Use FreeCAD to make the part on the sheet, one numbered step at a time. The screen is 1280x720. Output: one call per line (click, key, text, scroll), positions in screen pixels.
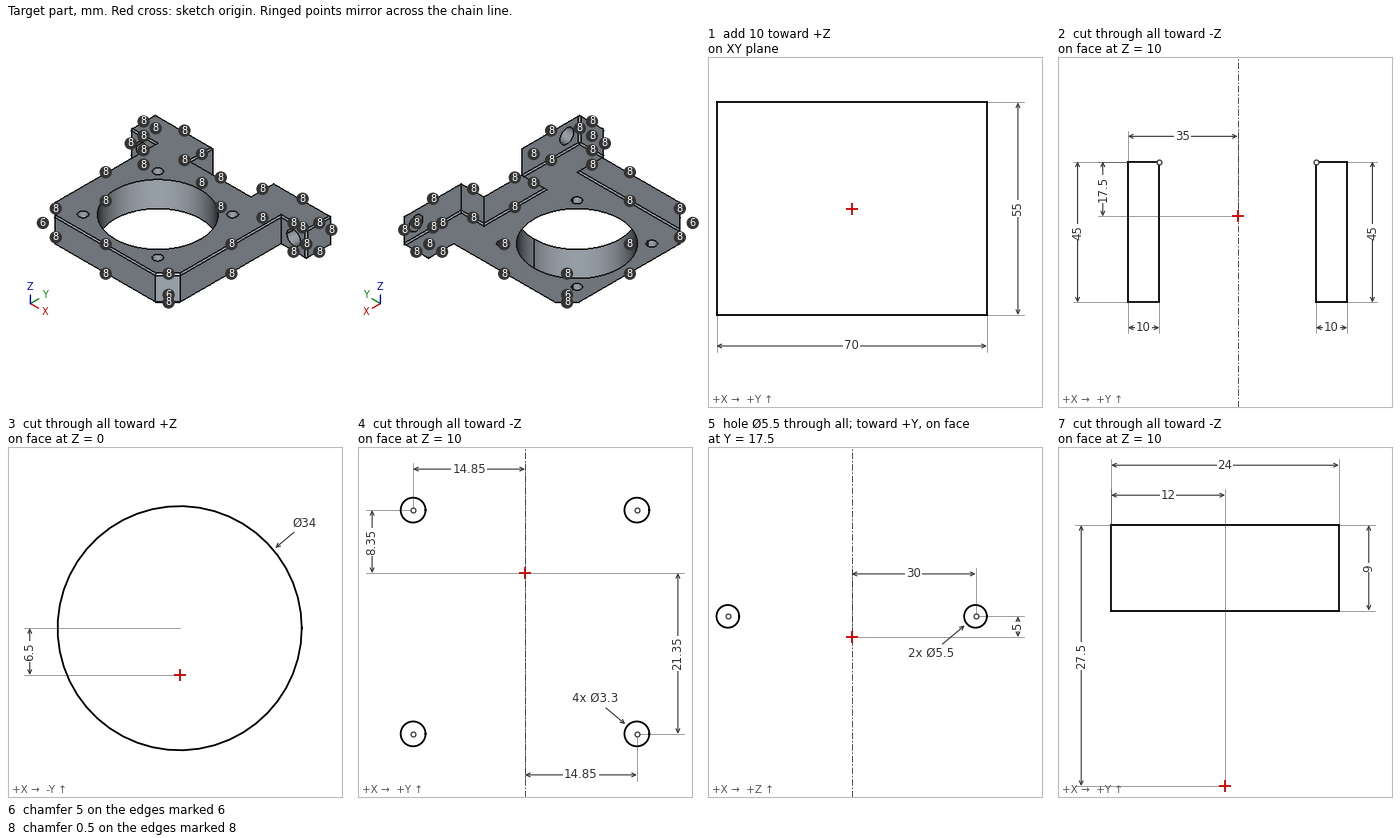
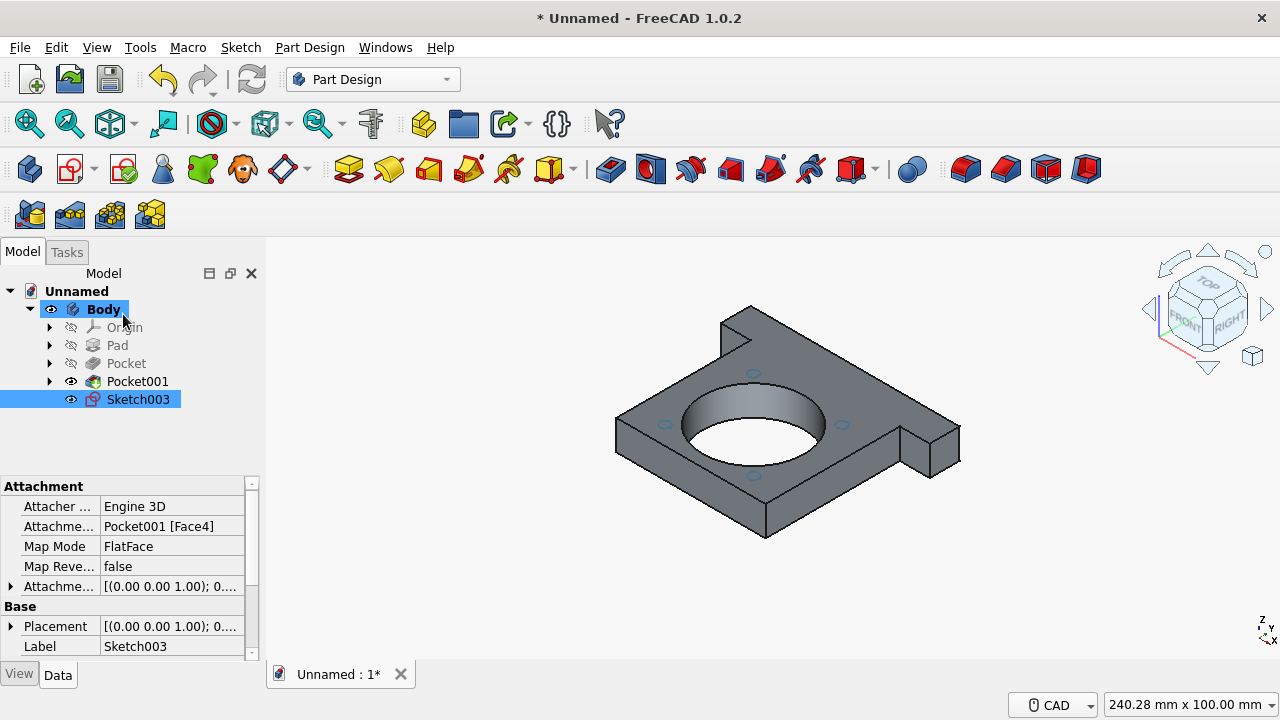
click(612, 170)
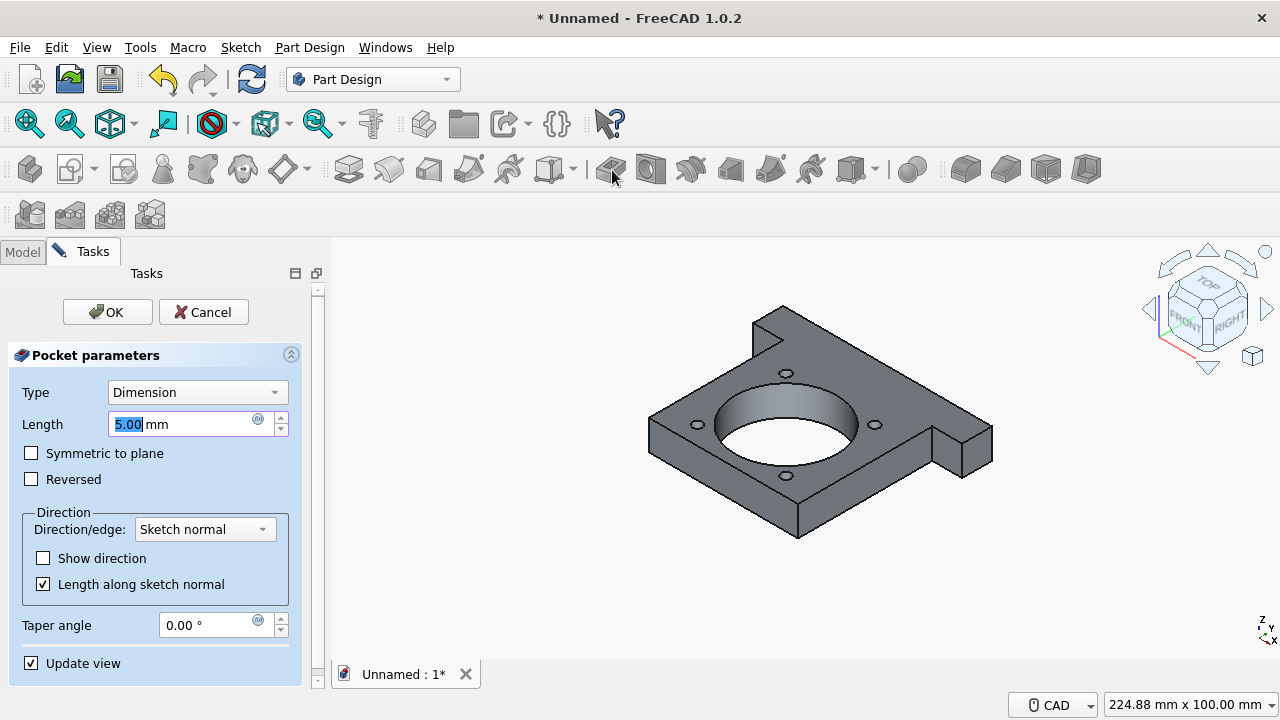
click(198, 392)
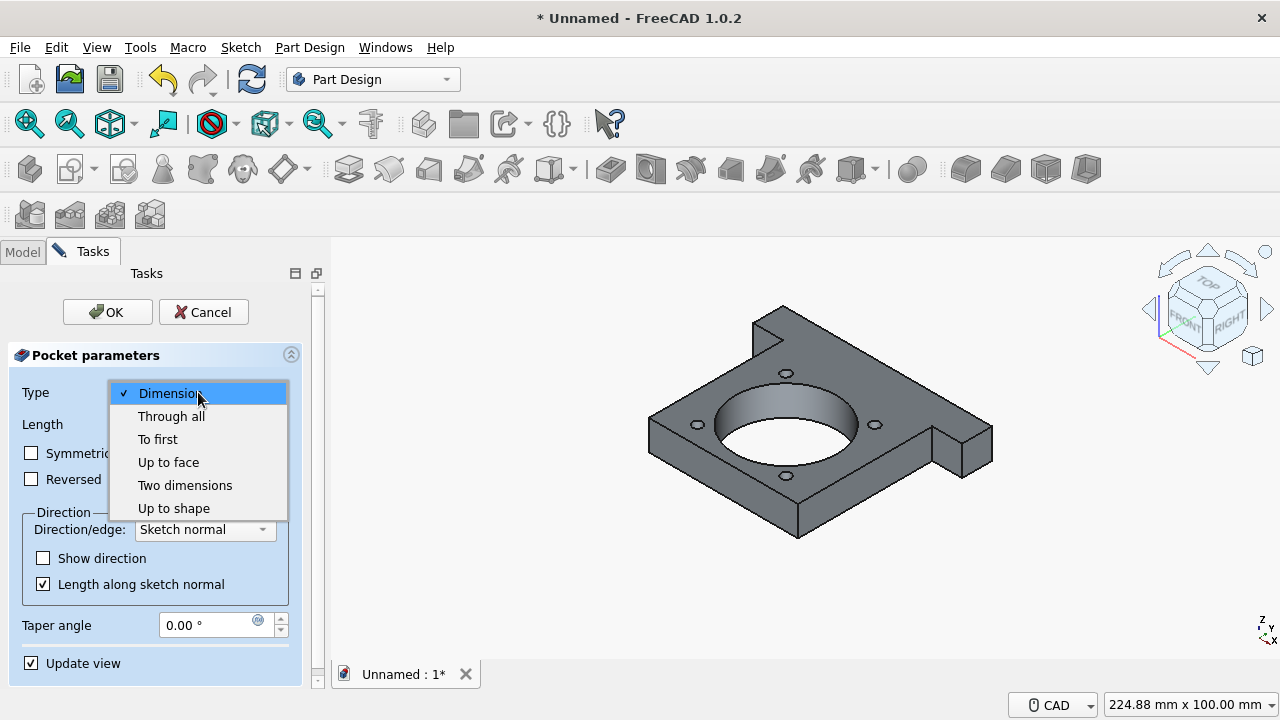
click(198, 416)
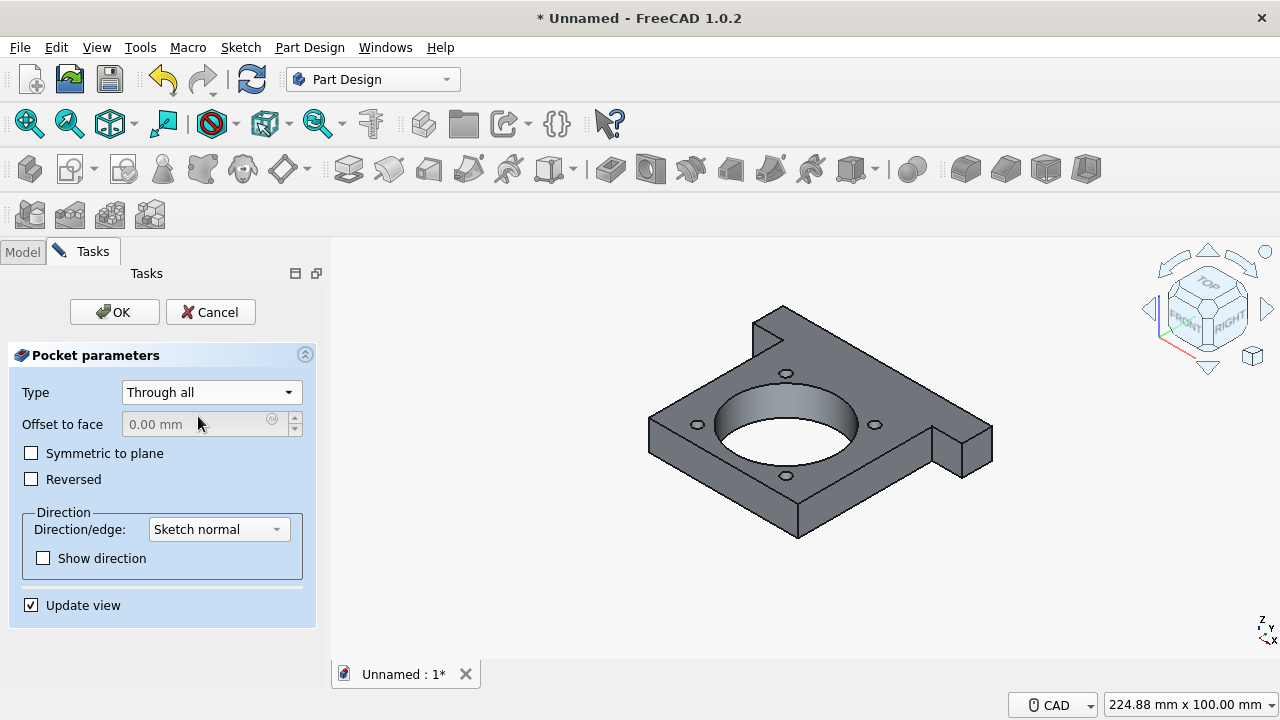
click(115, 312)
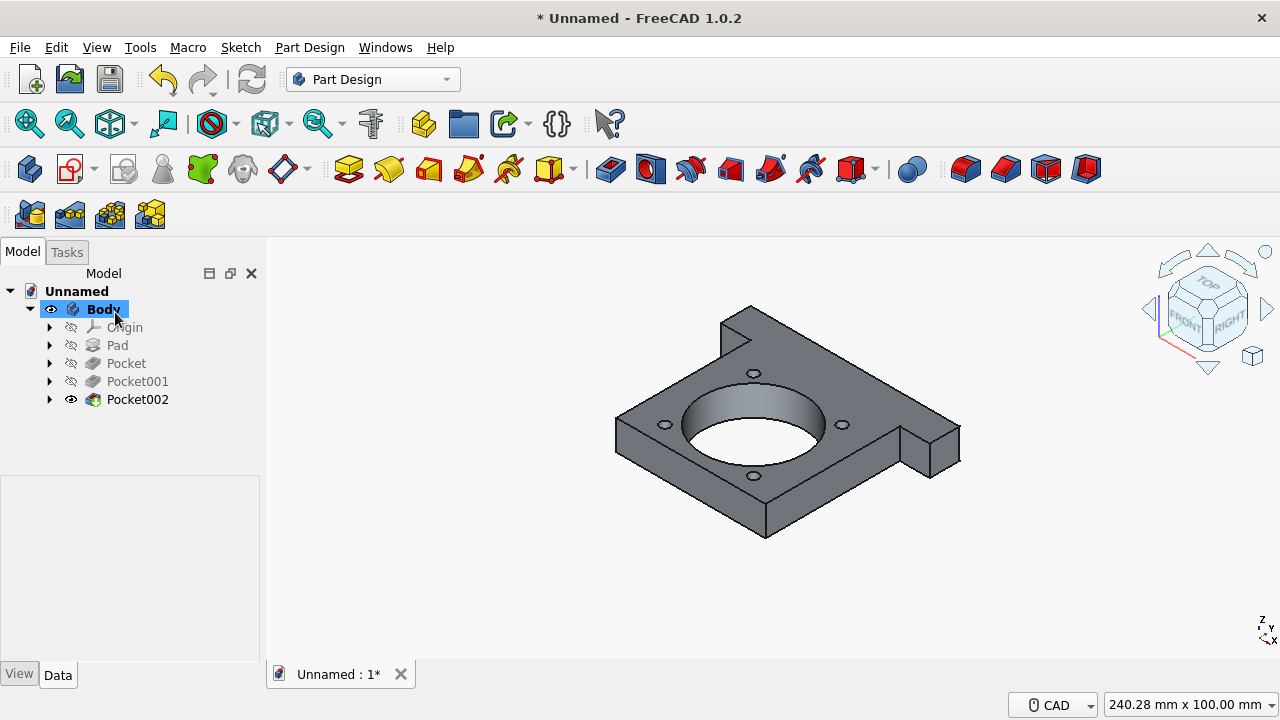
click(915, 451)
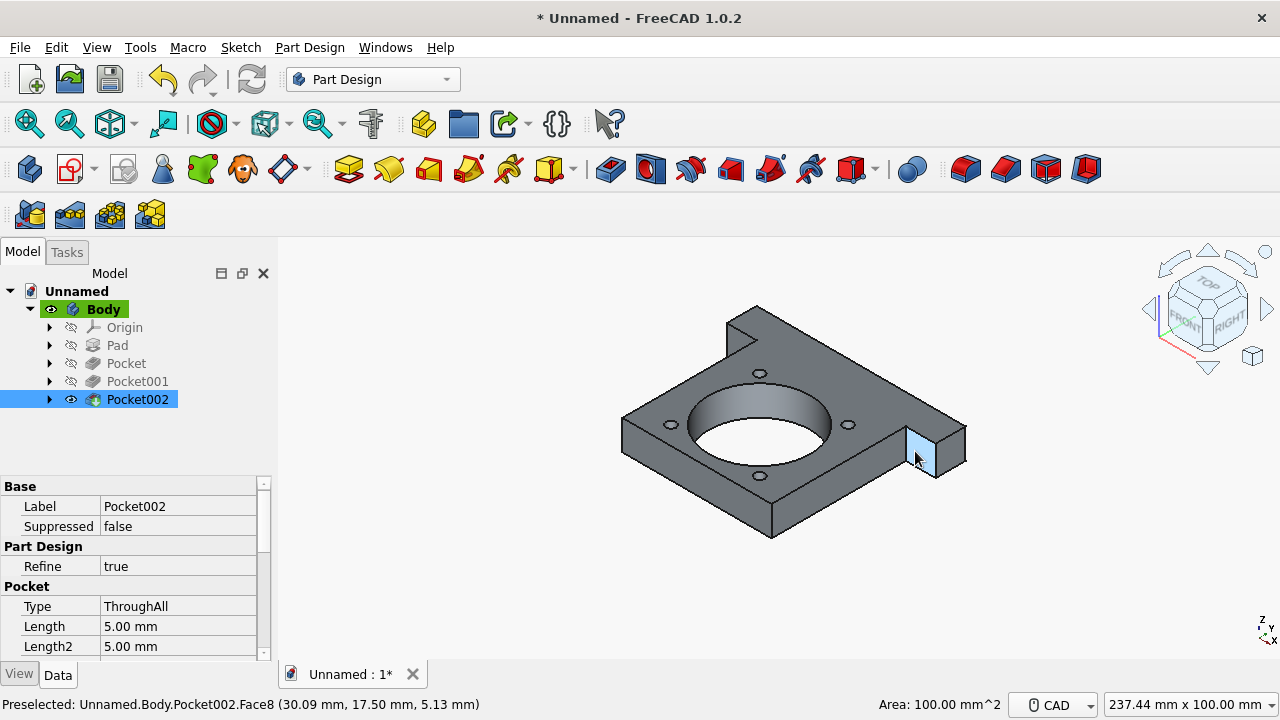
click(70, 170)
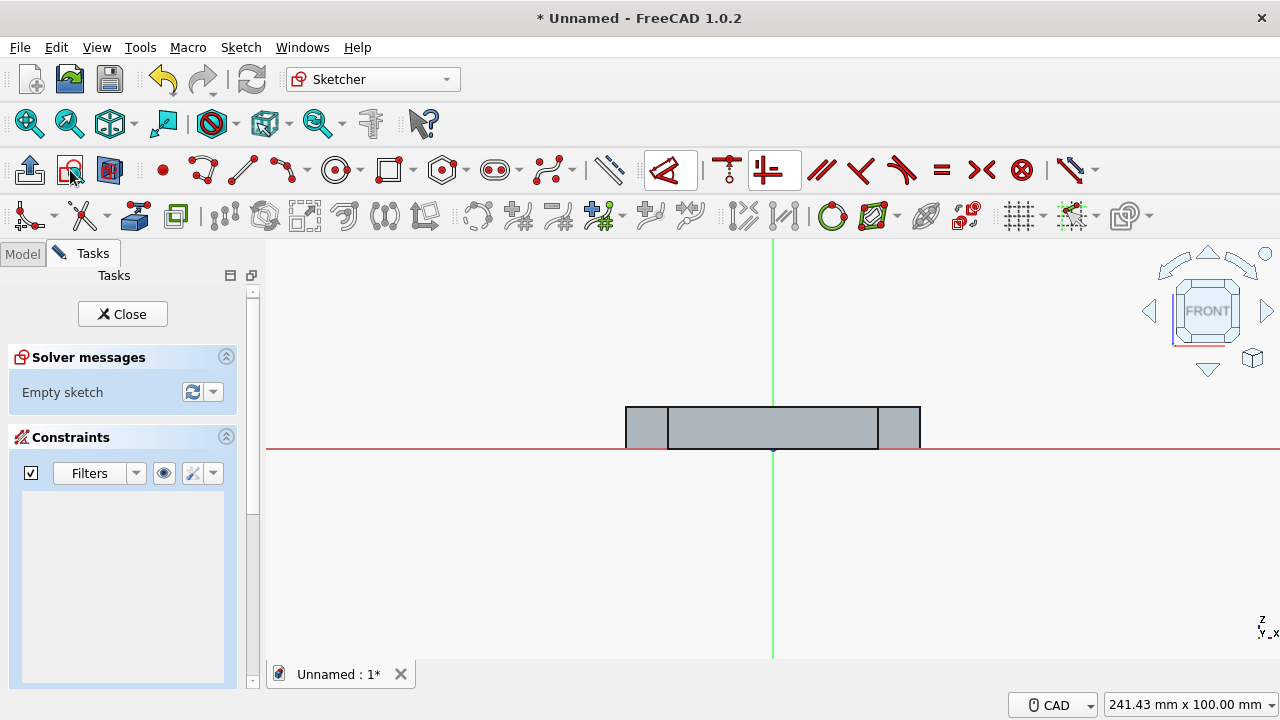
scroll(829, 419, up, 4)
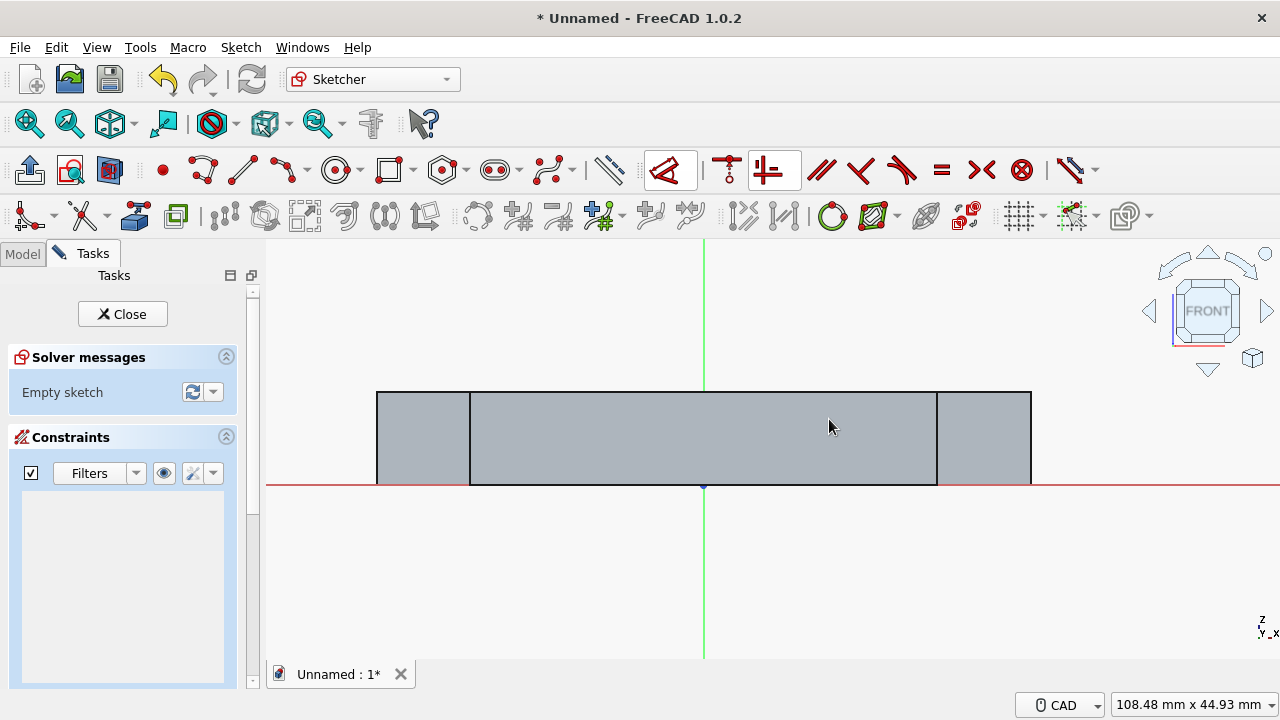
key(g)
key(c)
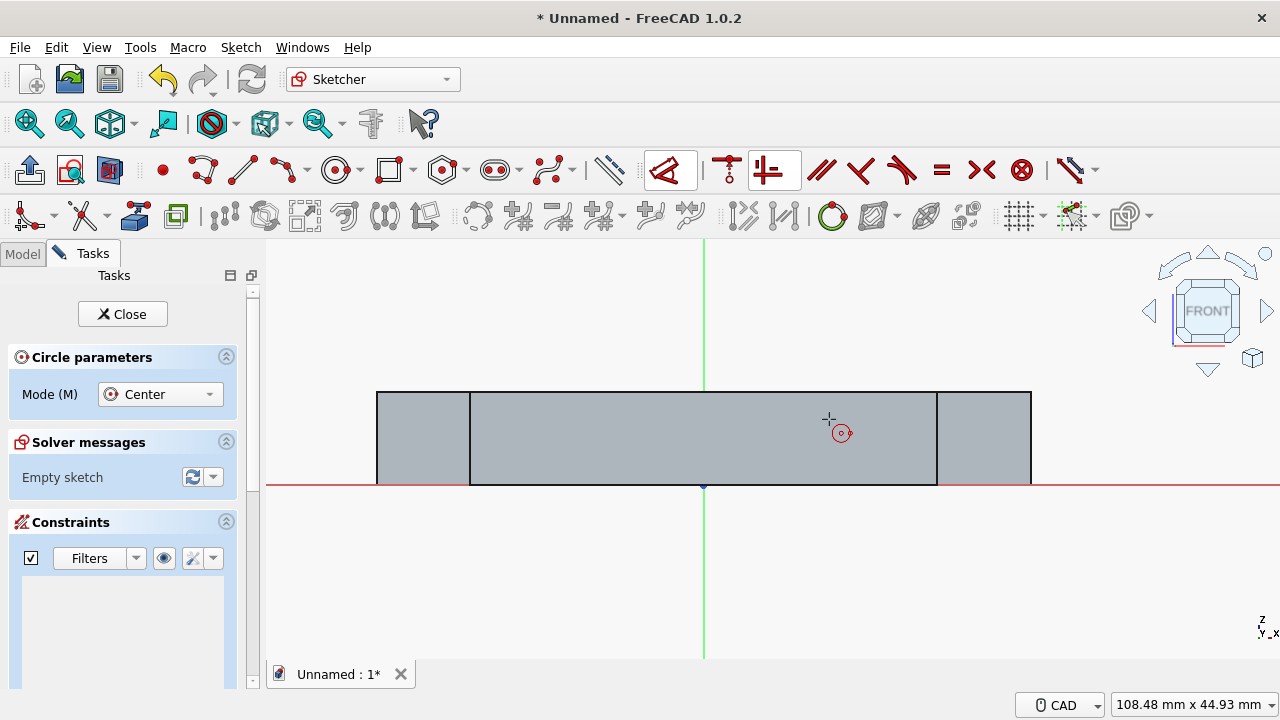
click(984, 439)
move(1002, 420)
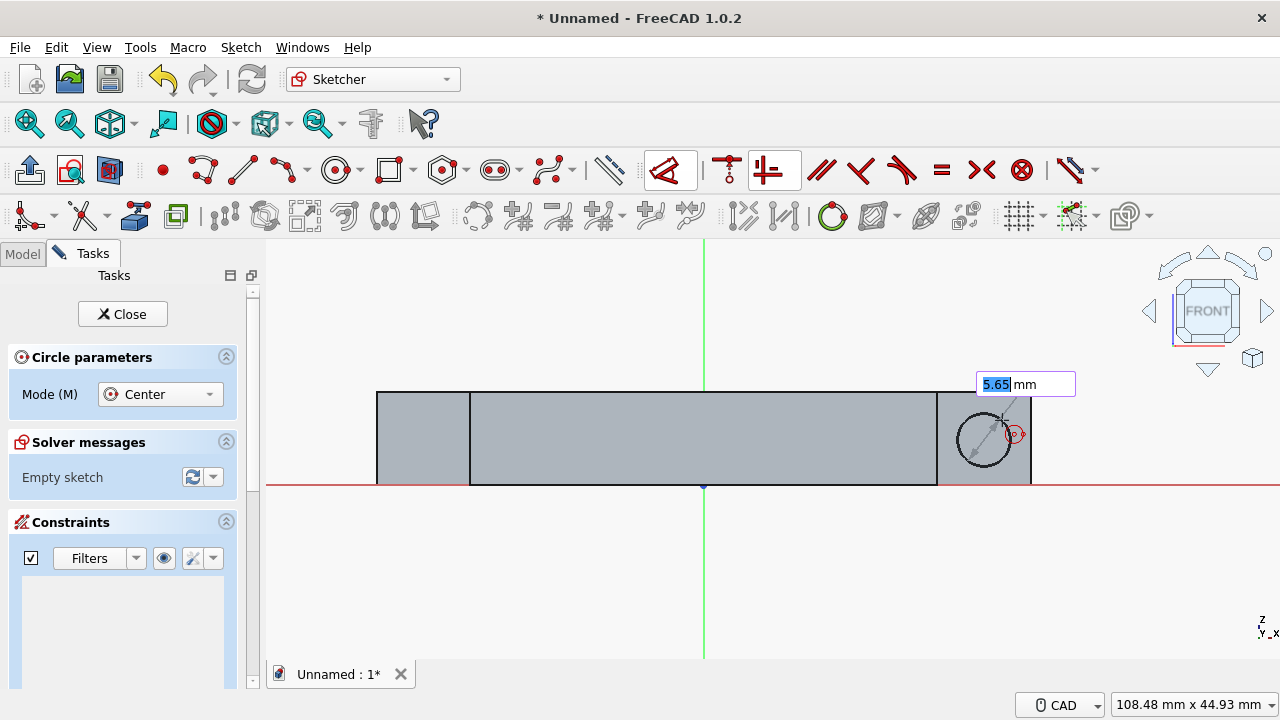
text(5.5)
key(Return)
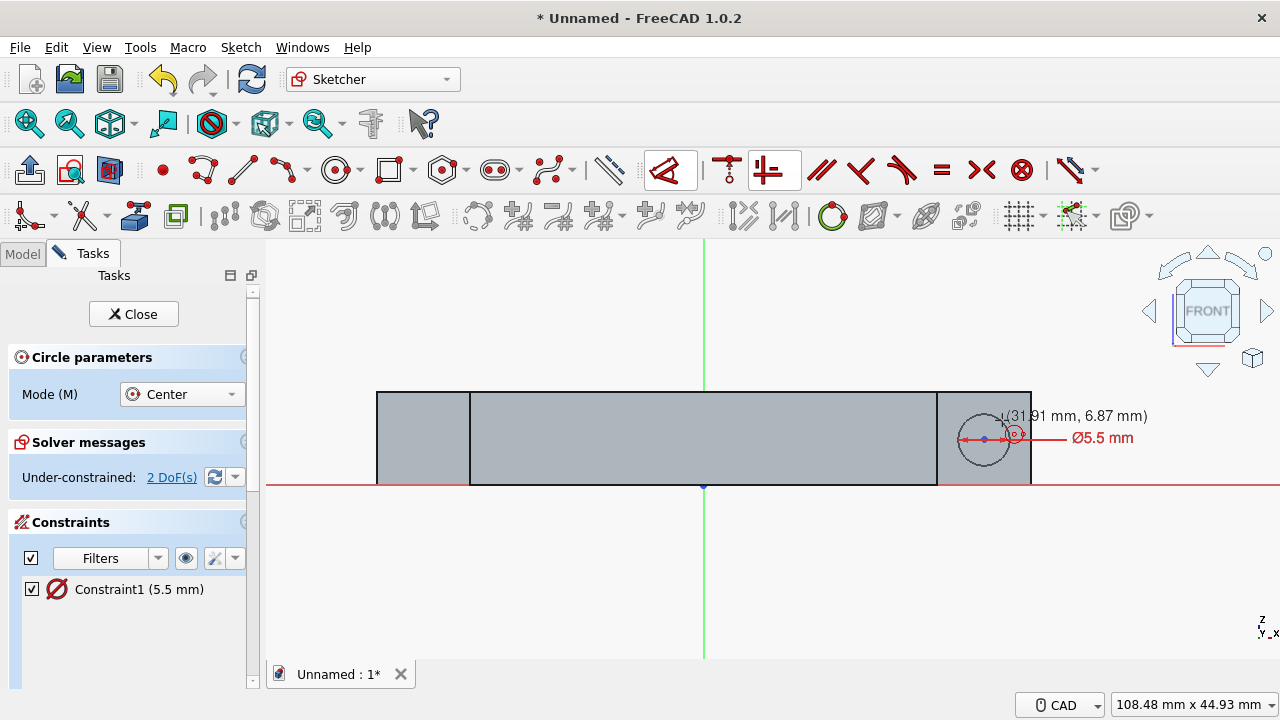
click(423, 439)
move(441, 420)